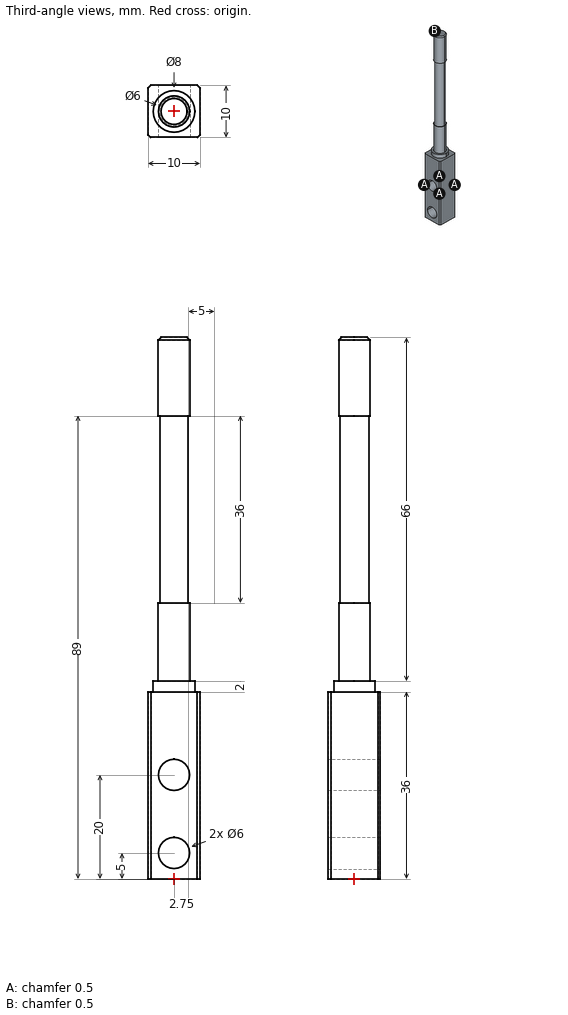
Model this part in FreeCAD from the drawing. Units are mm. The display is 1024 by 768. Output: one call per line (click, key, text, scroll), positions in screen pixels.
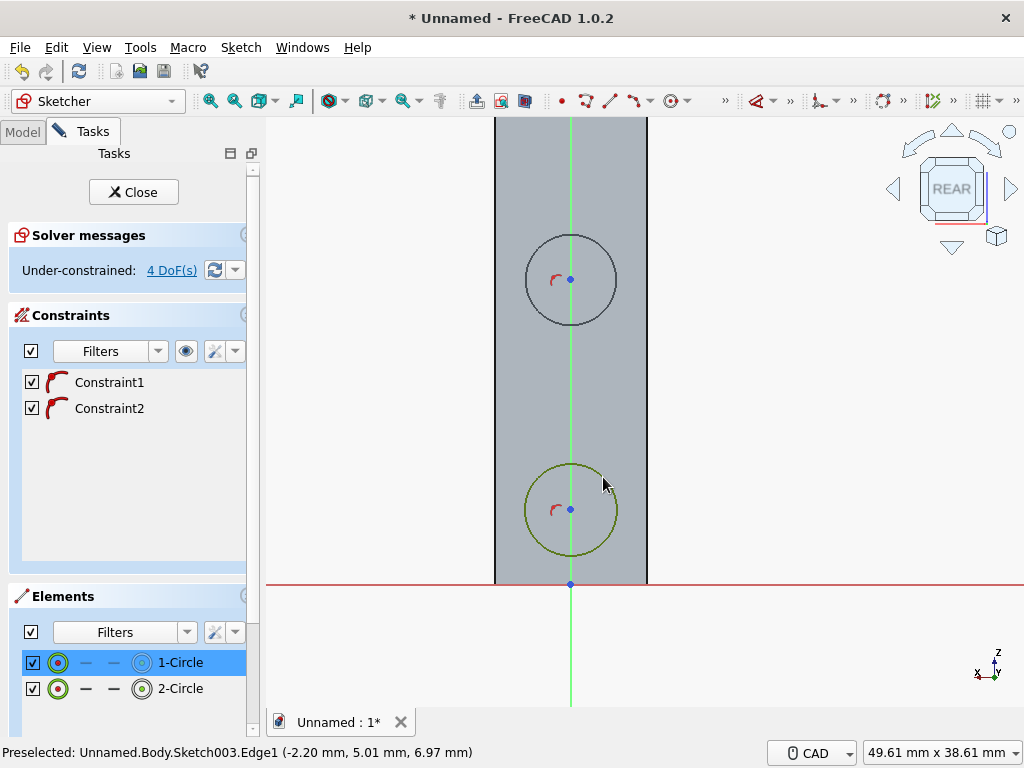
click(603, 248)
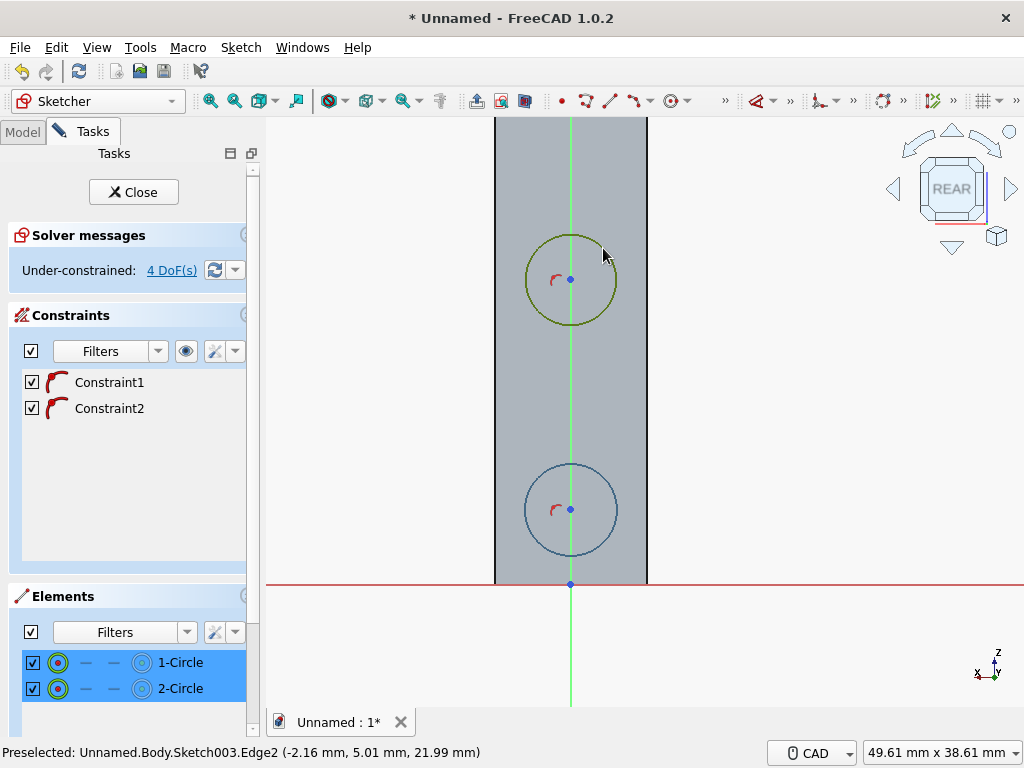
key(e)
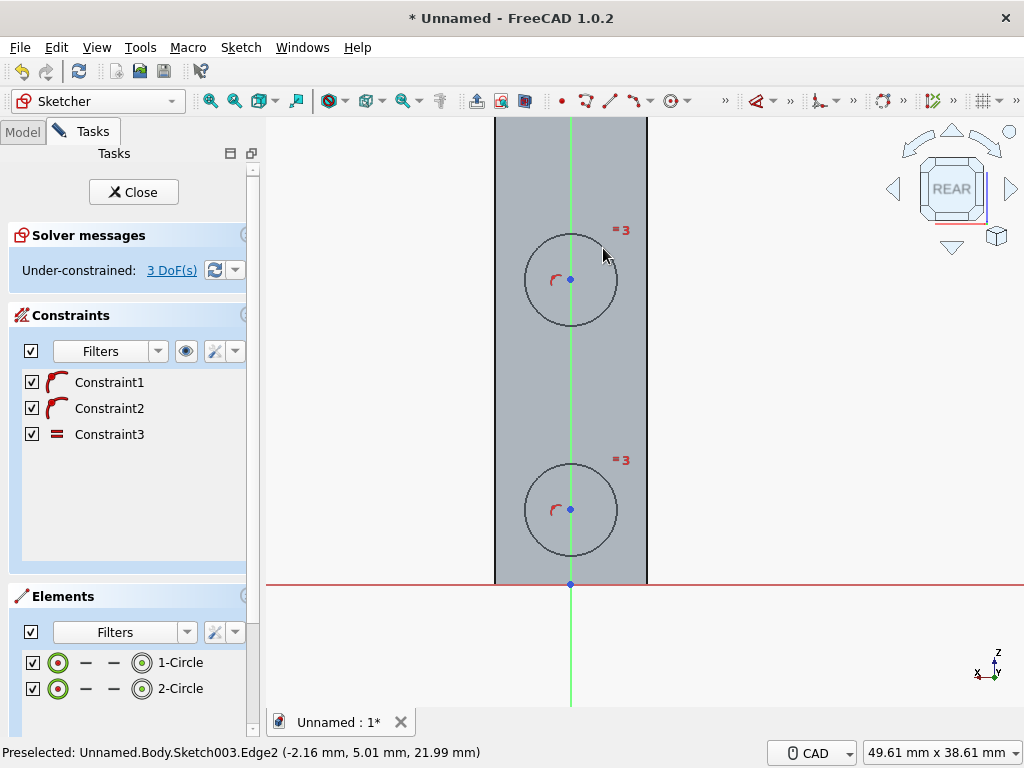
key(d)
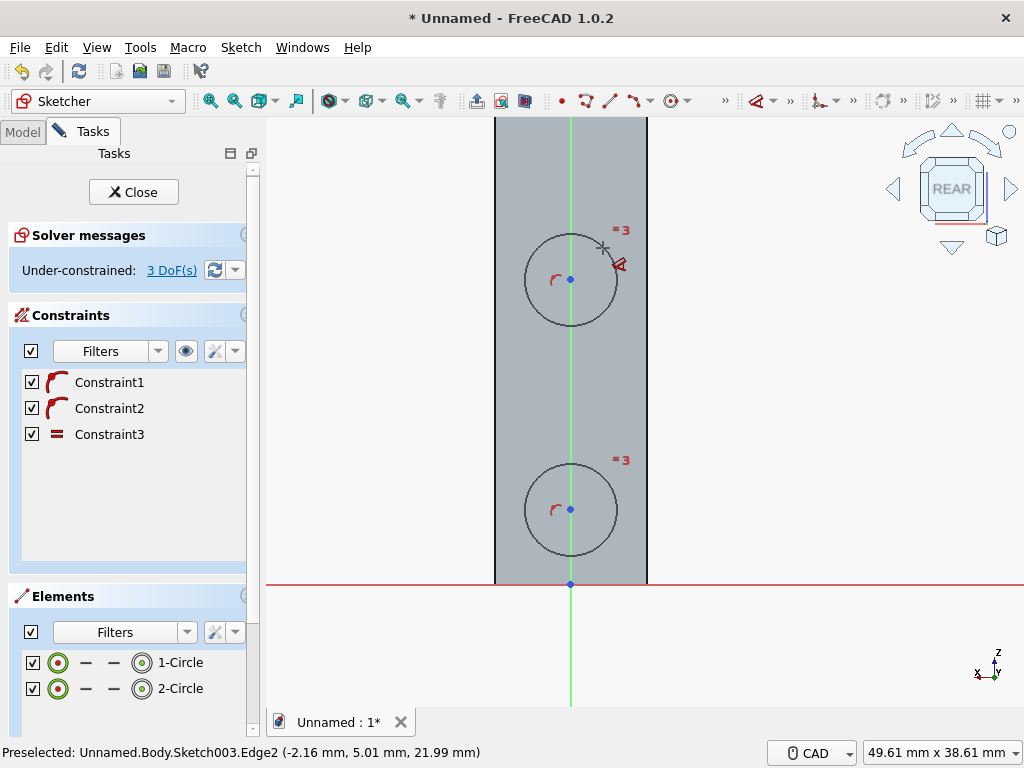
click(603, 477)
click(625, 454)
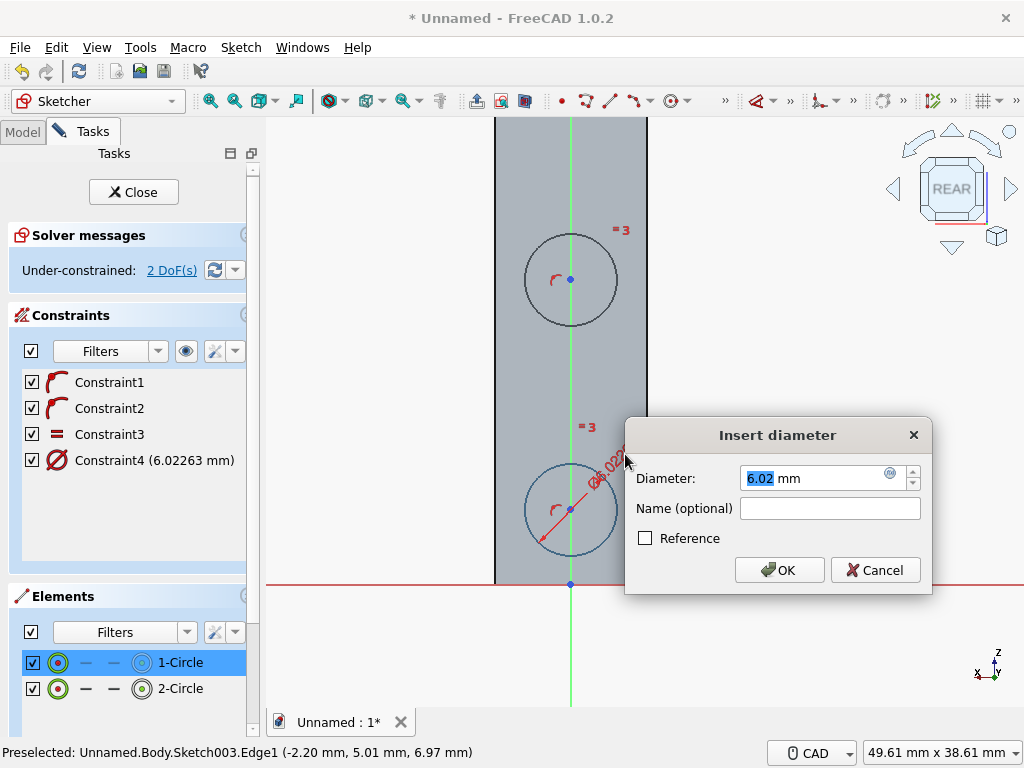
text(6)
key(Return)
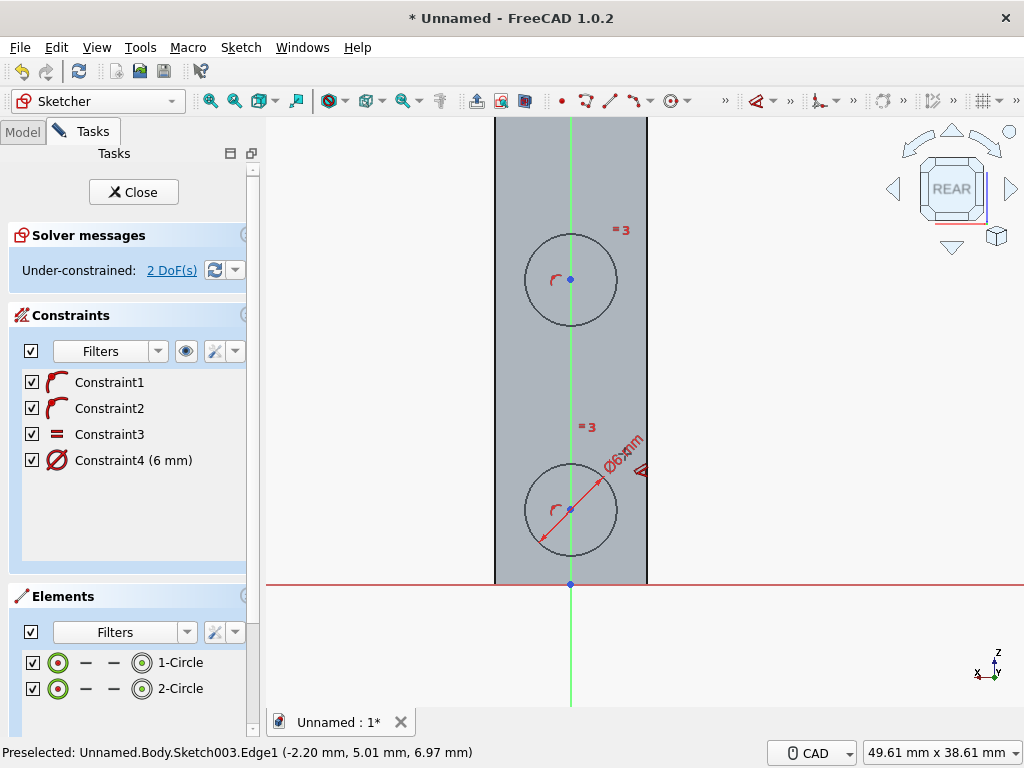
click(571, 510)
click(605, 565)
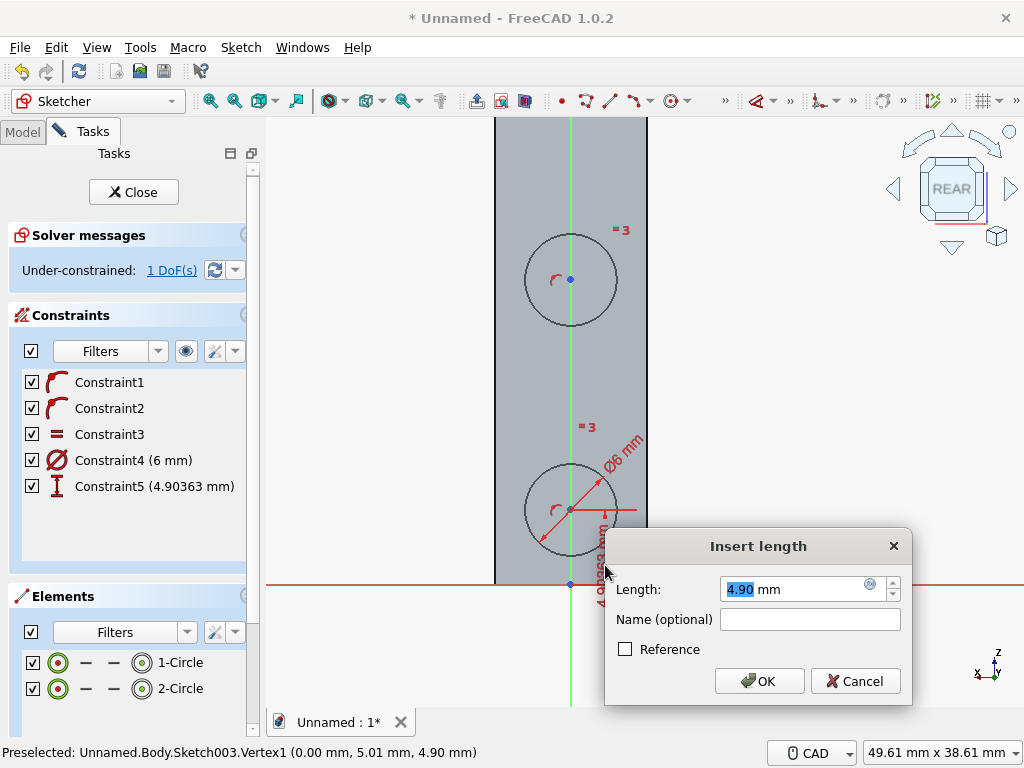
text(5)
key(Return)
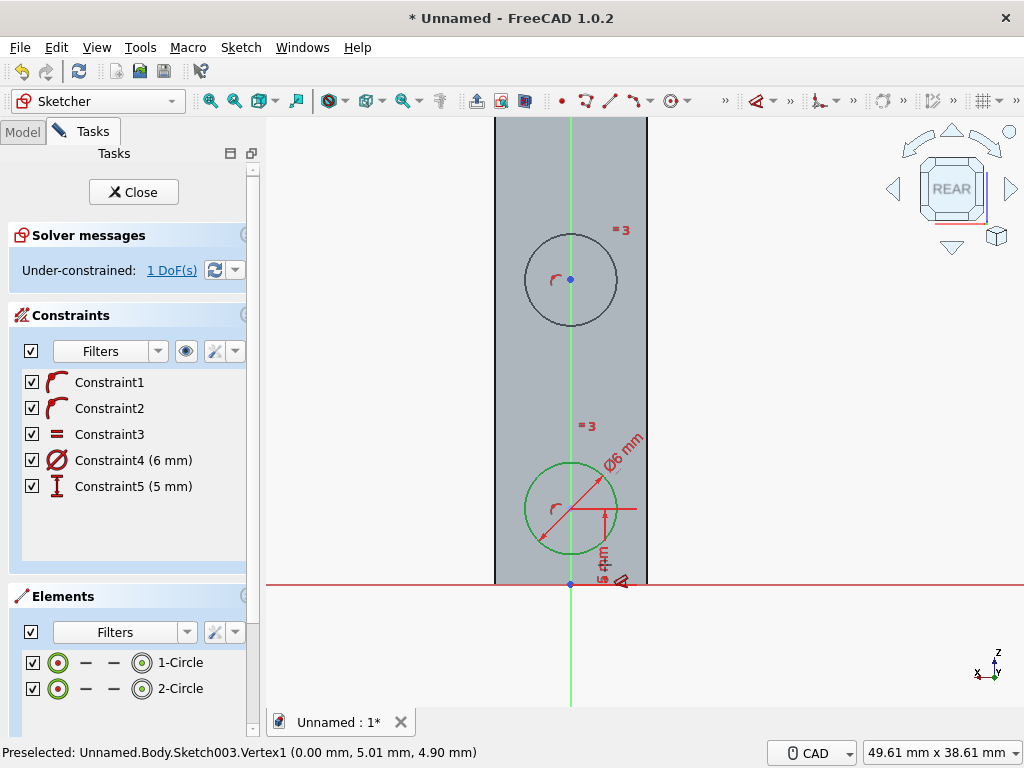
click(571, 280)
click(605, 432)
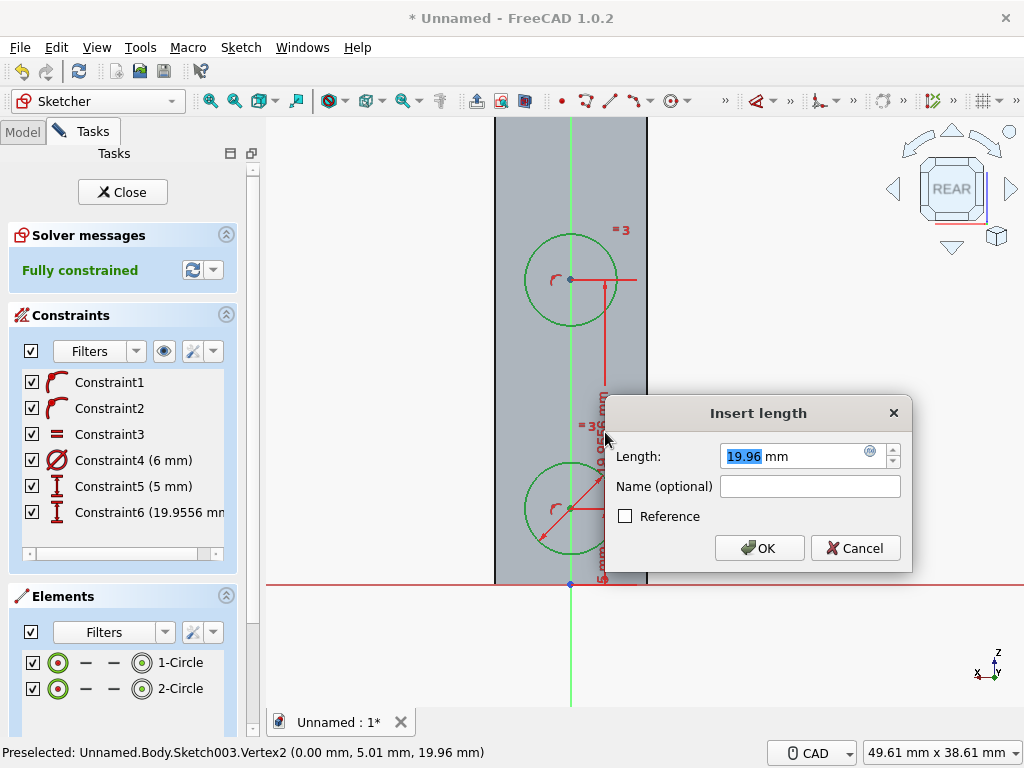
text(20)
key(Return)
key(Escape)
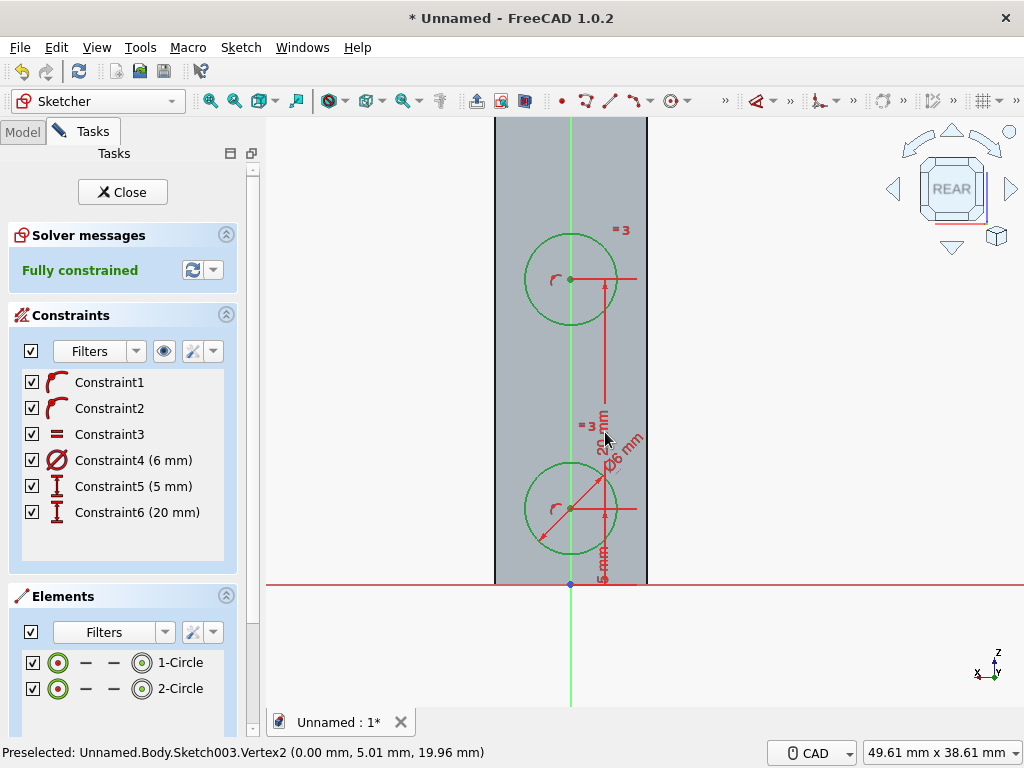
click(123, 192)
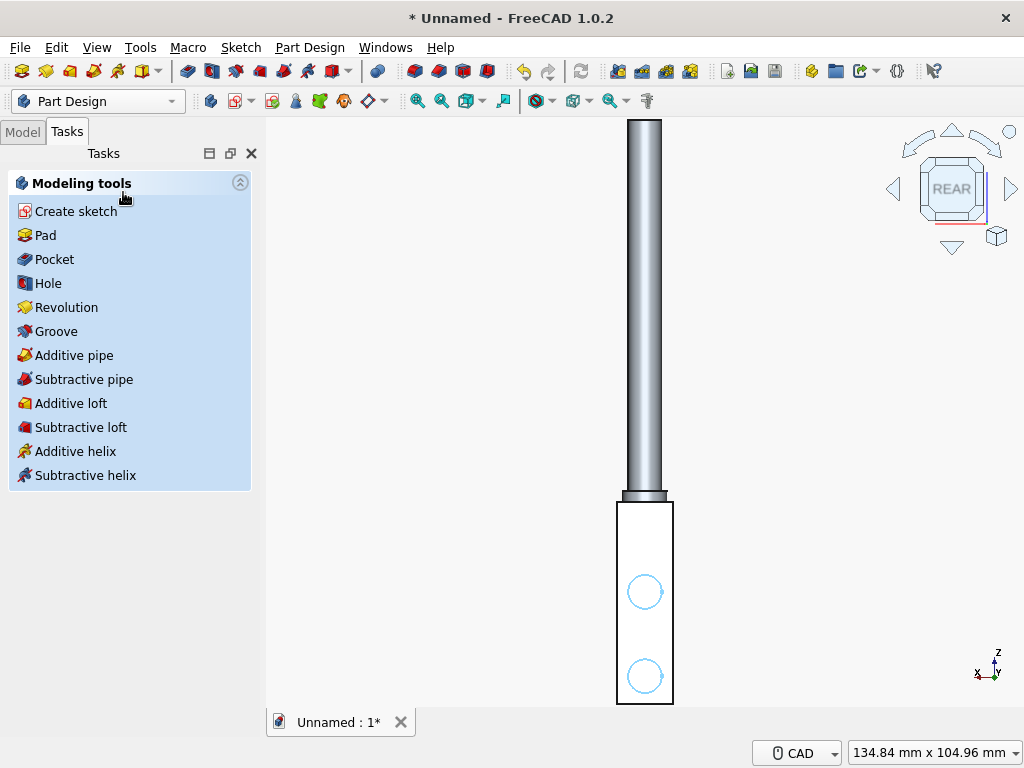
click(188, 72)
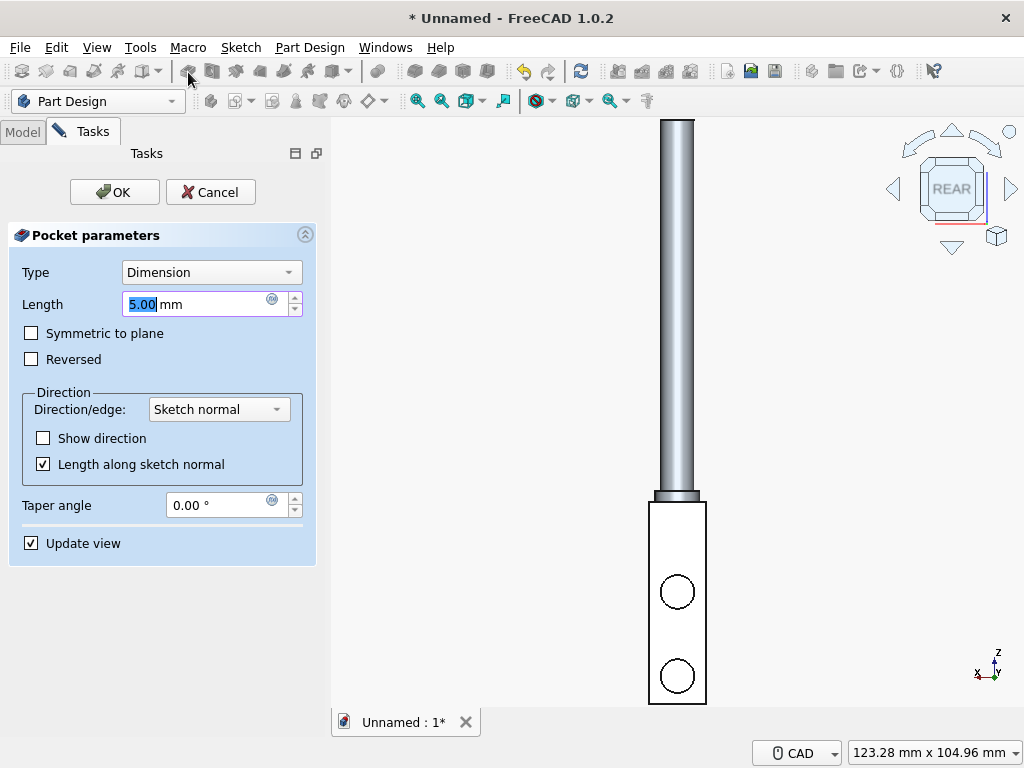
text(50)
key(Tab)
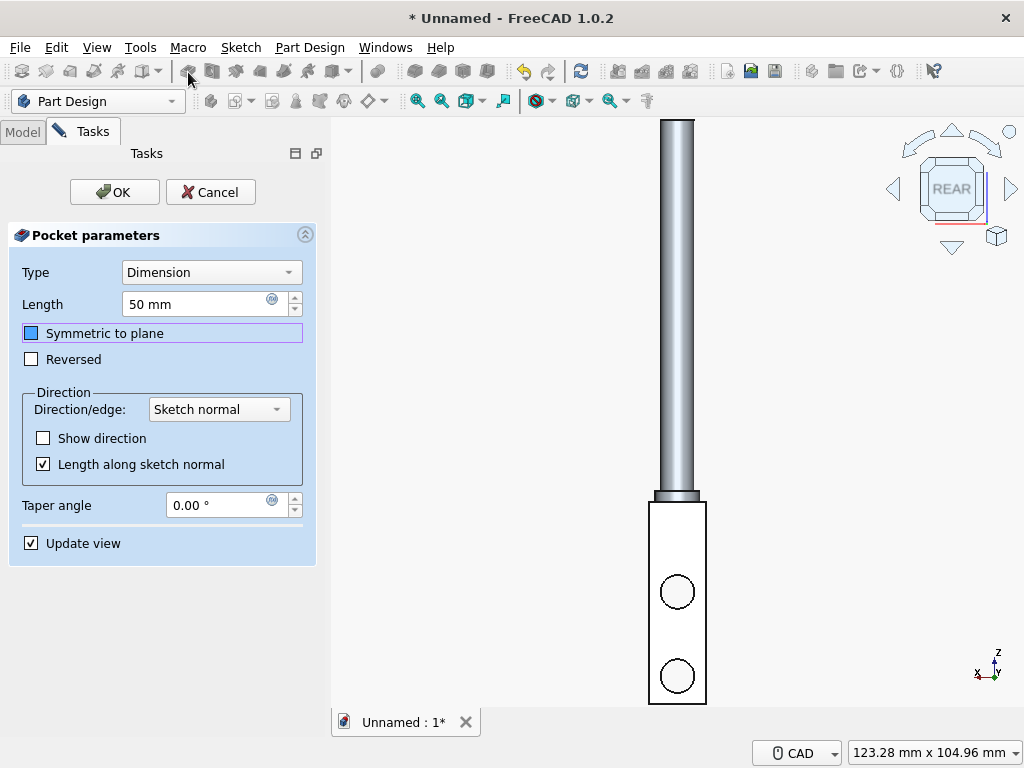
click(115, 192)